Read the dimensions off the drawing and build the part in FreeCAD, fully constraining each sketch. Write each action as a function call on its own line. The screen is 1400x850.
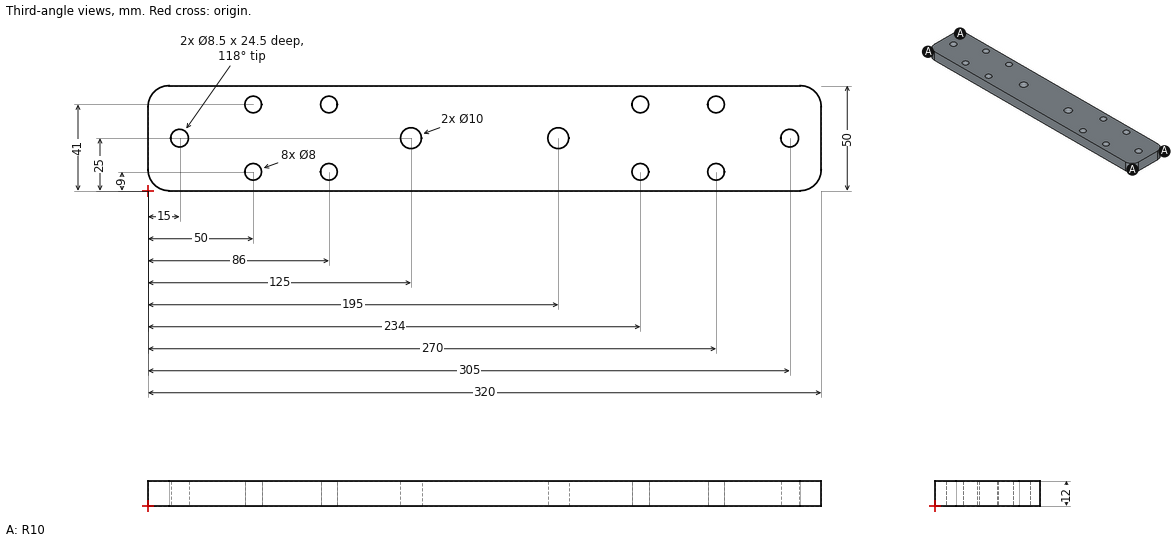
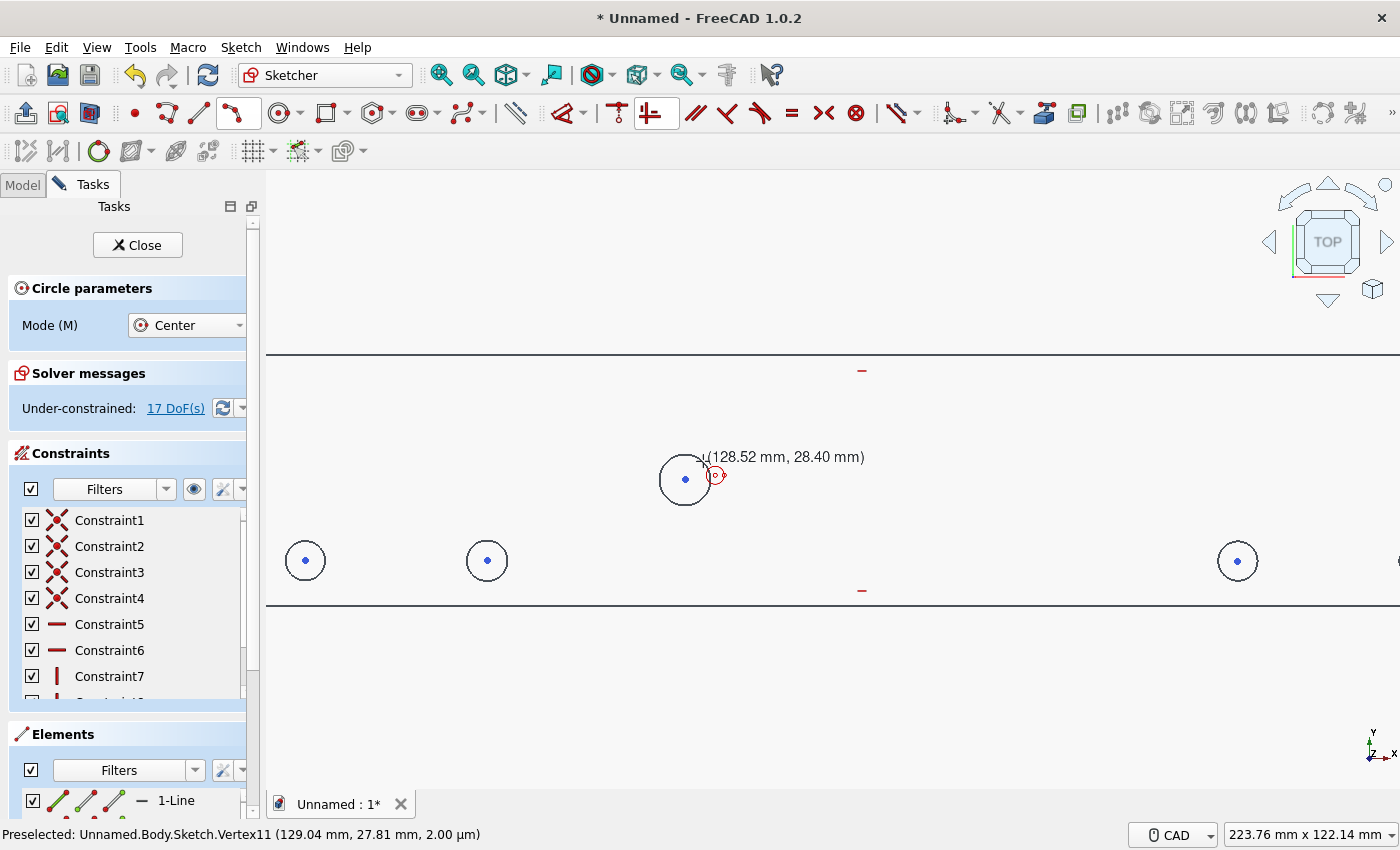
click(305, 398)
click(319, 384)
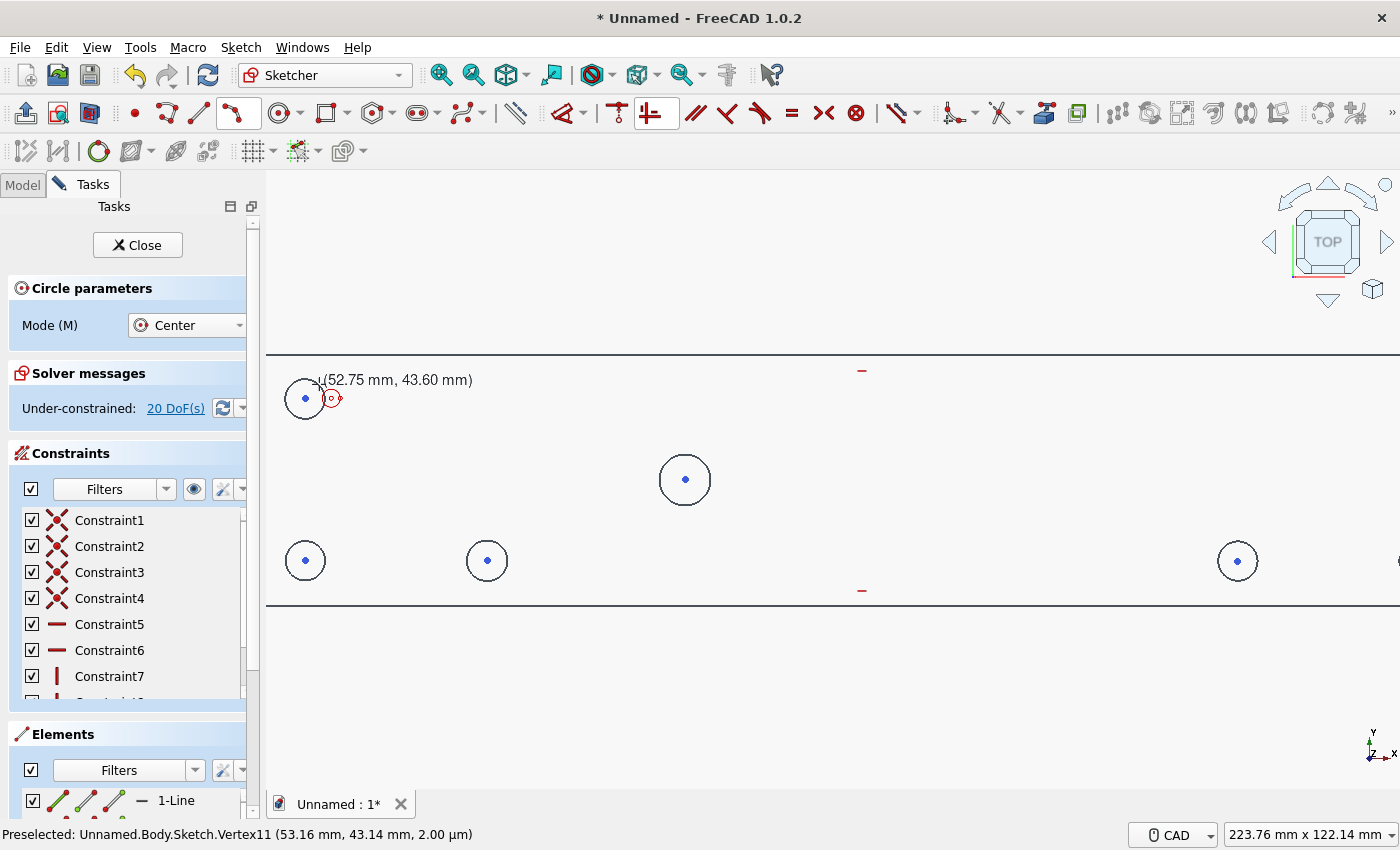
click(487, 398)
click(502, 384)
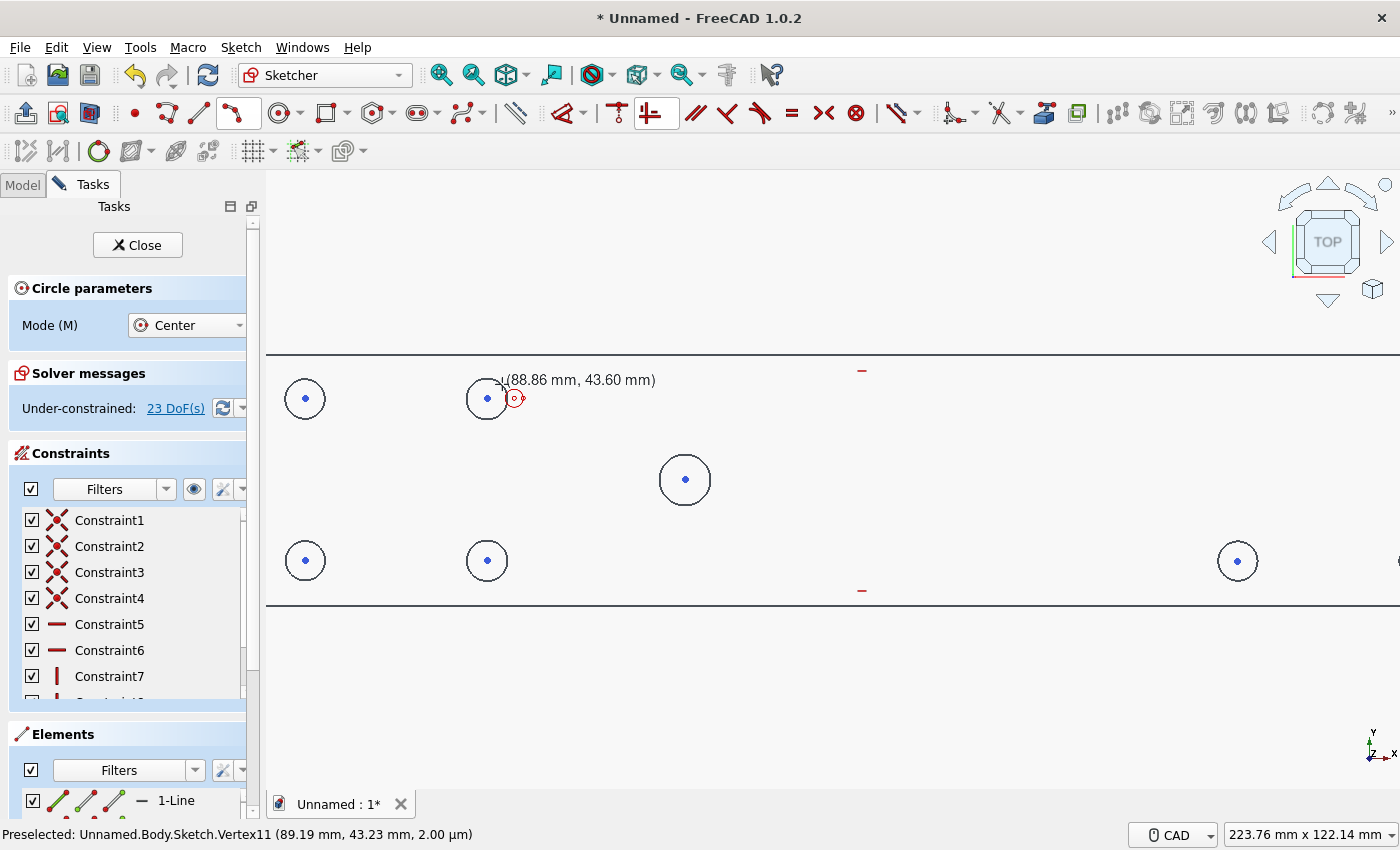
click(1040, 479)
click(1058, 461)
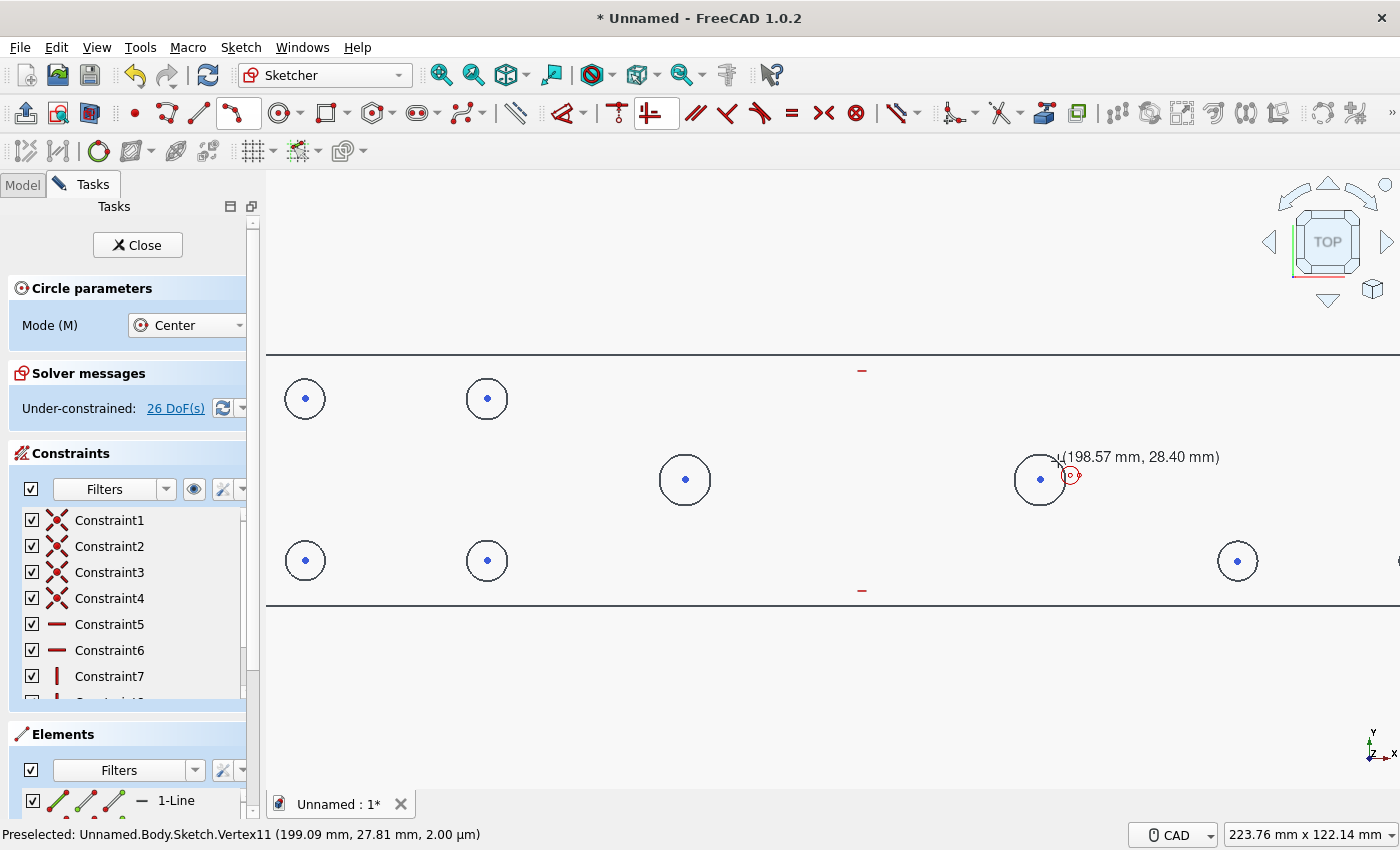
scroll(685, 480, down, 4)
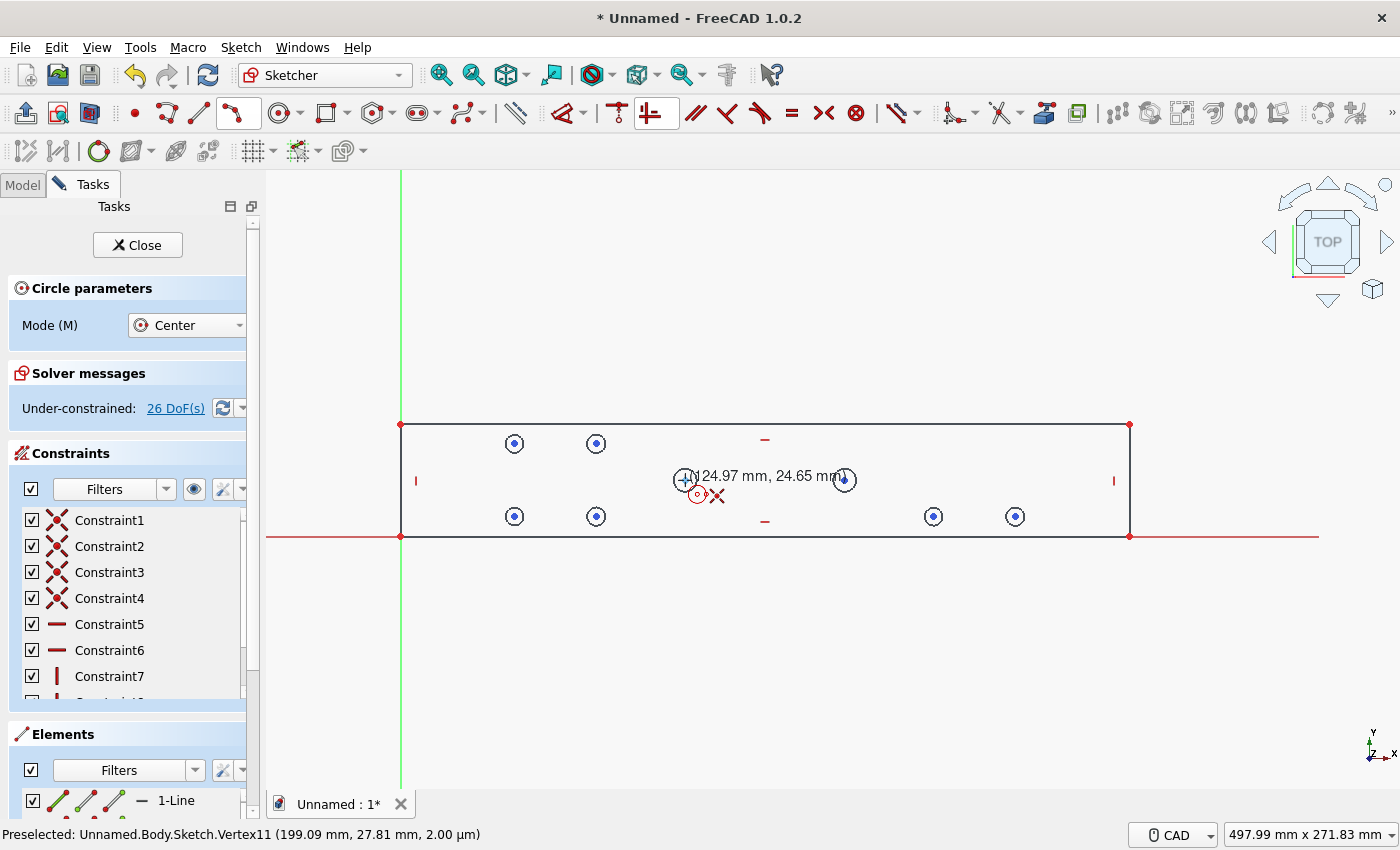
scroll(933, 444, up, 5)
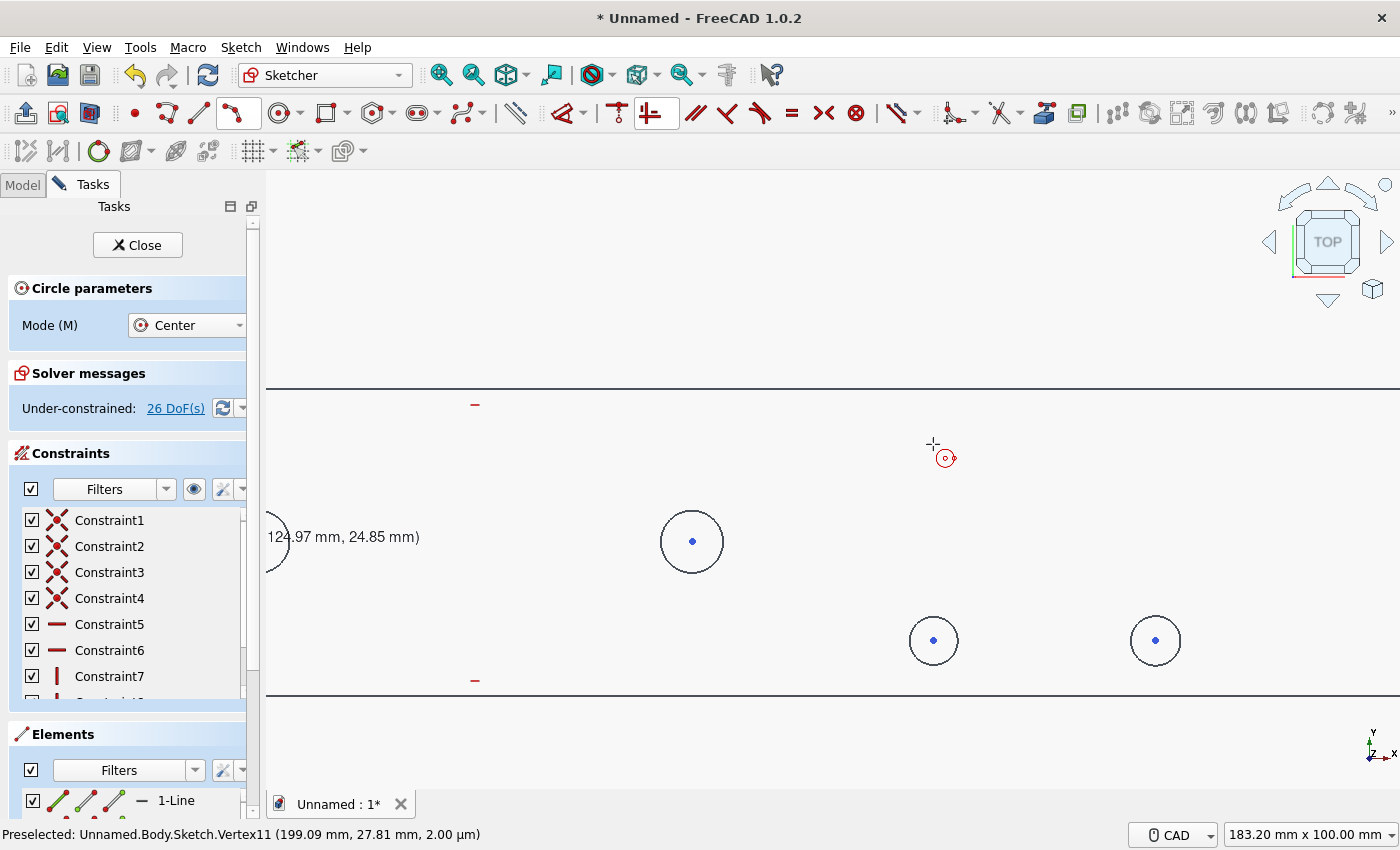
click(933, 442)
click(951, 424)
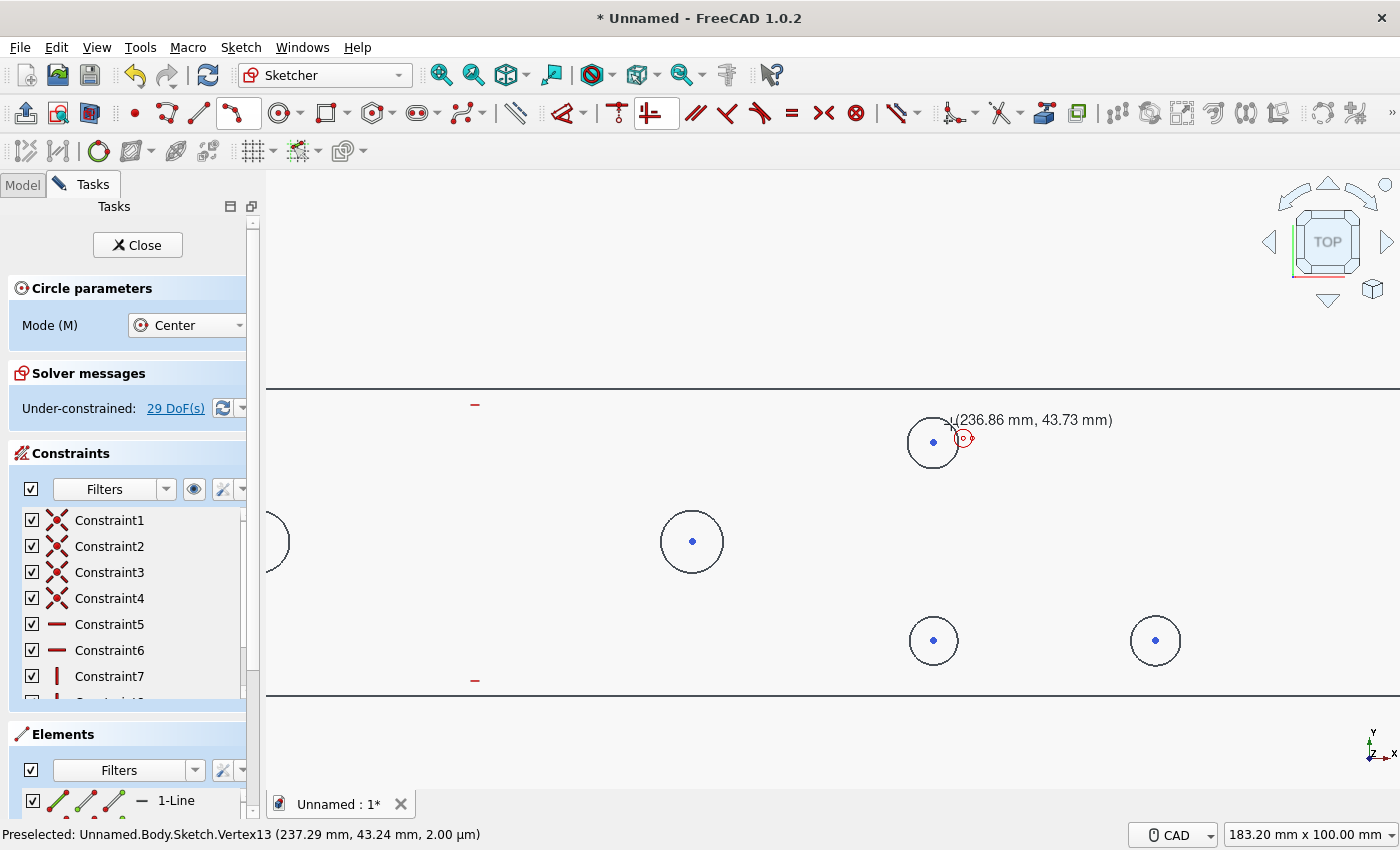
click(1156, 442)
click(1174, 424)
key(Escape)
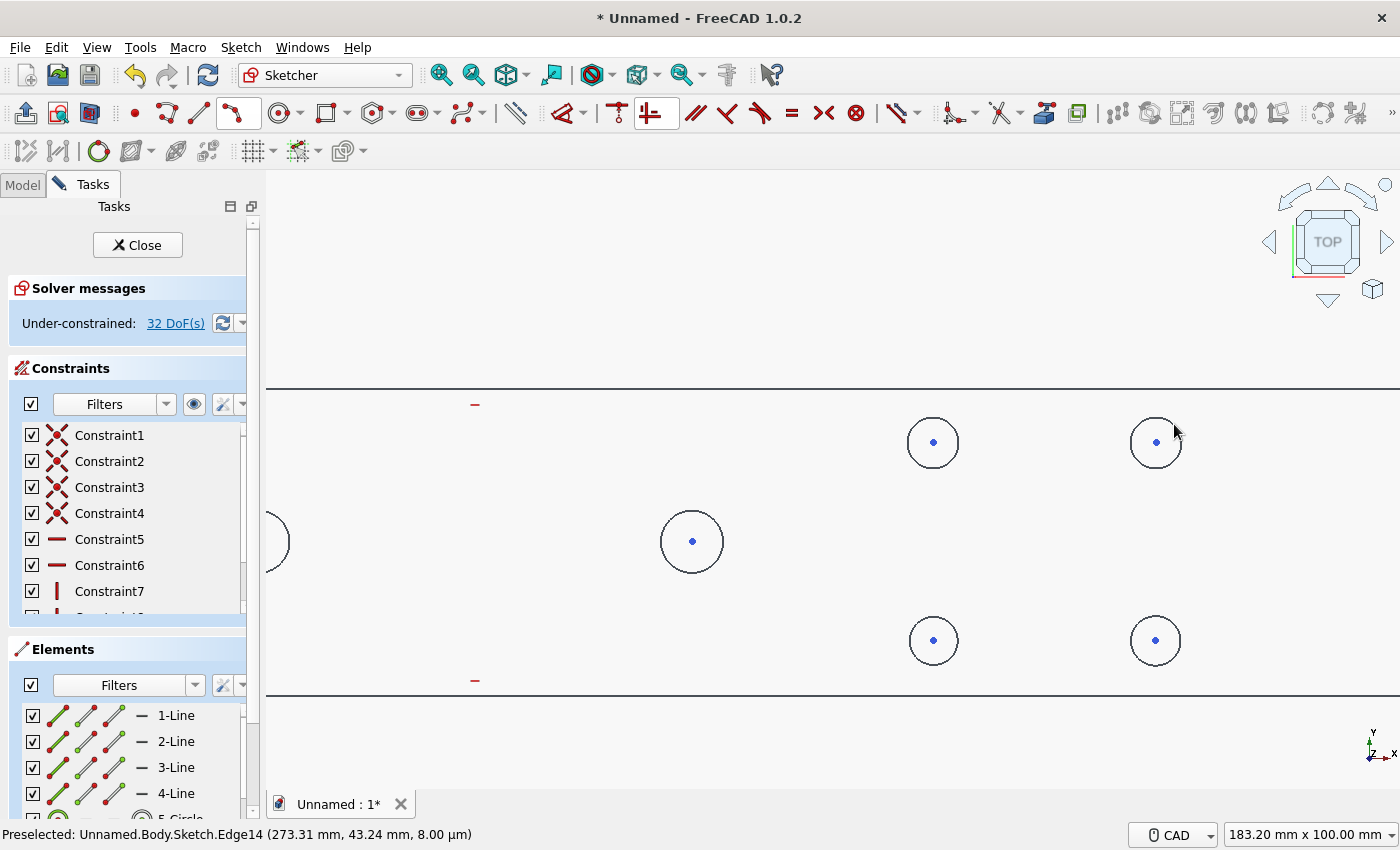
scroll(933, 444, down, 5)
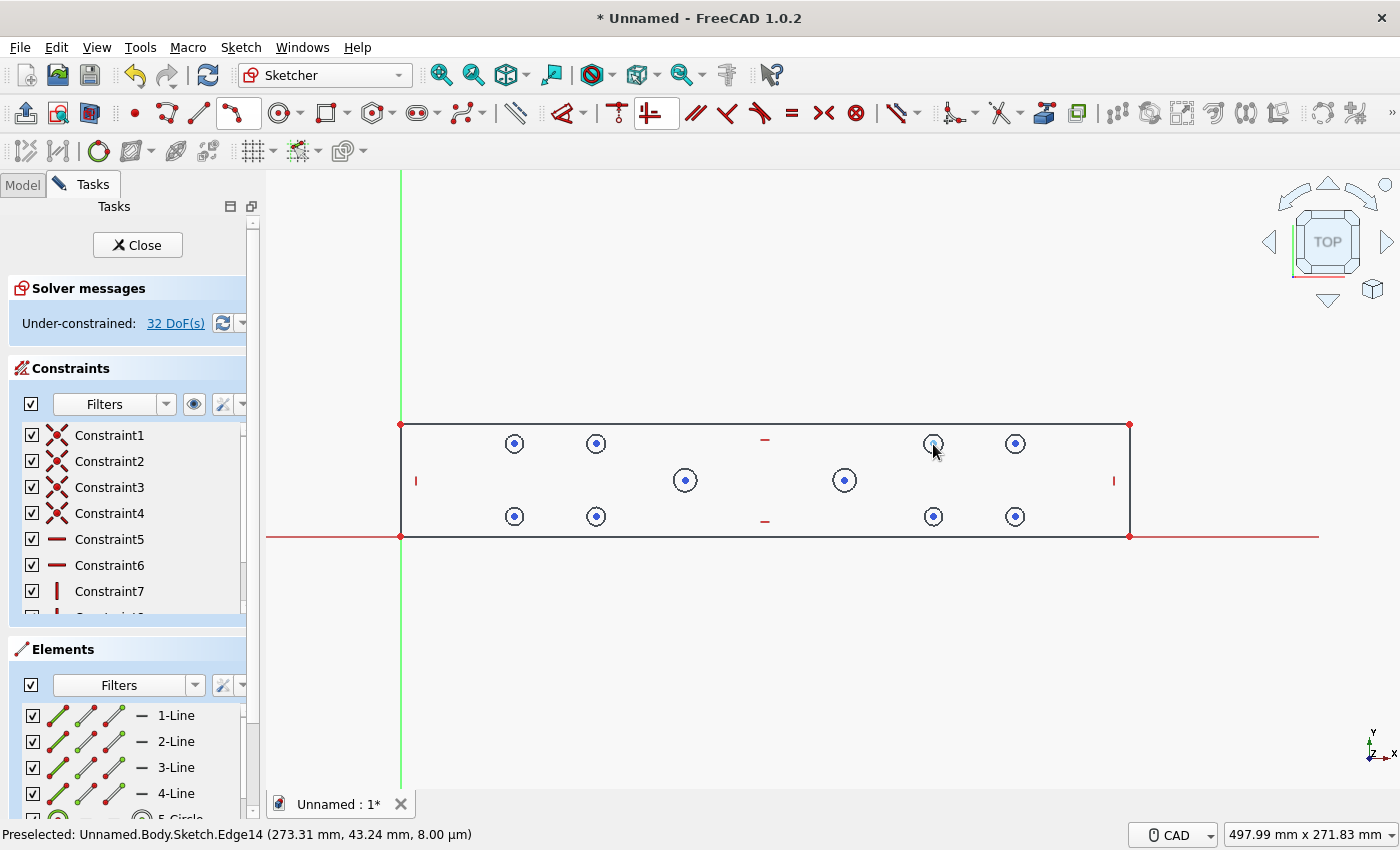
scroll(521, 510, up, 3)